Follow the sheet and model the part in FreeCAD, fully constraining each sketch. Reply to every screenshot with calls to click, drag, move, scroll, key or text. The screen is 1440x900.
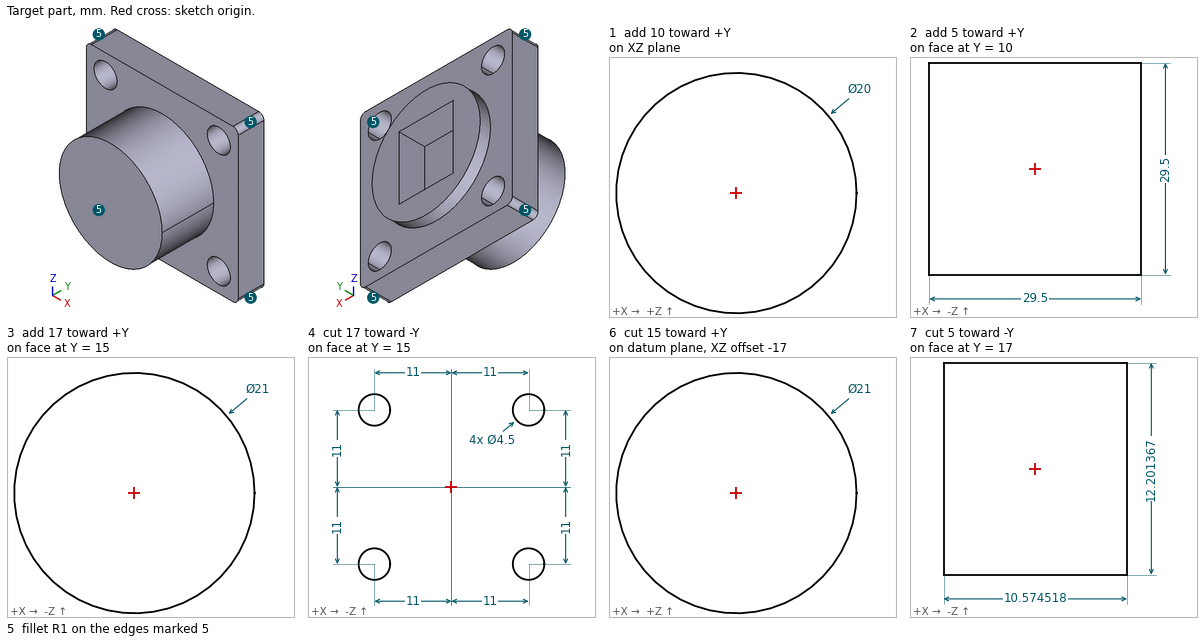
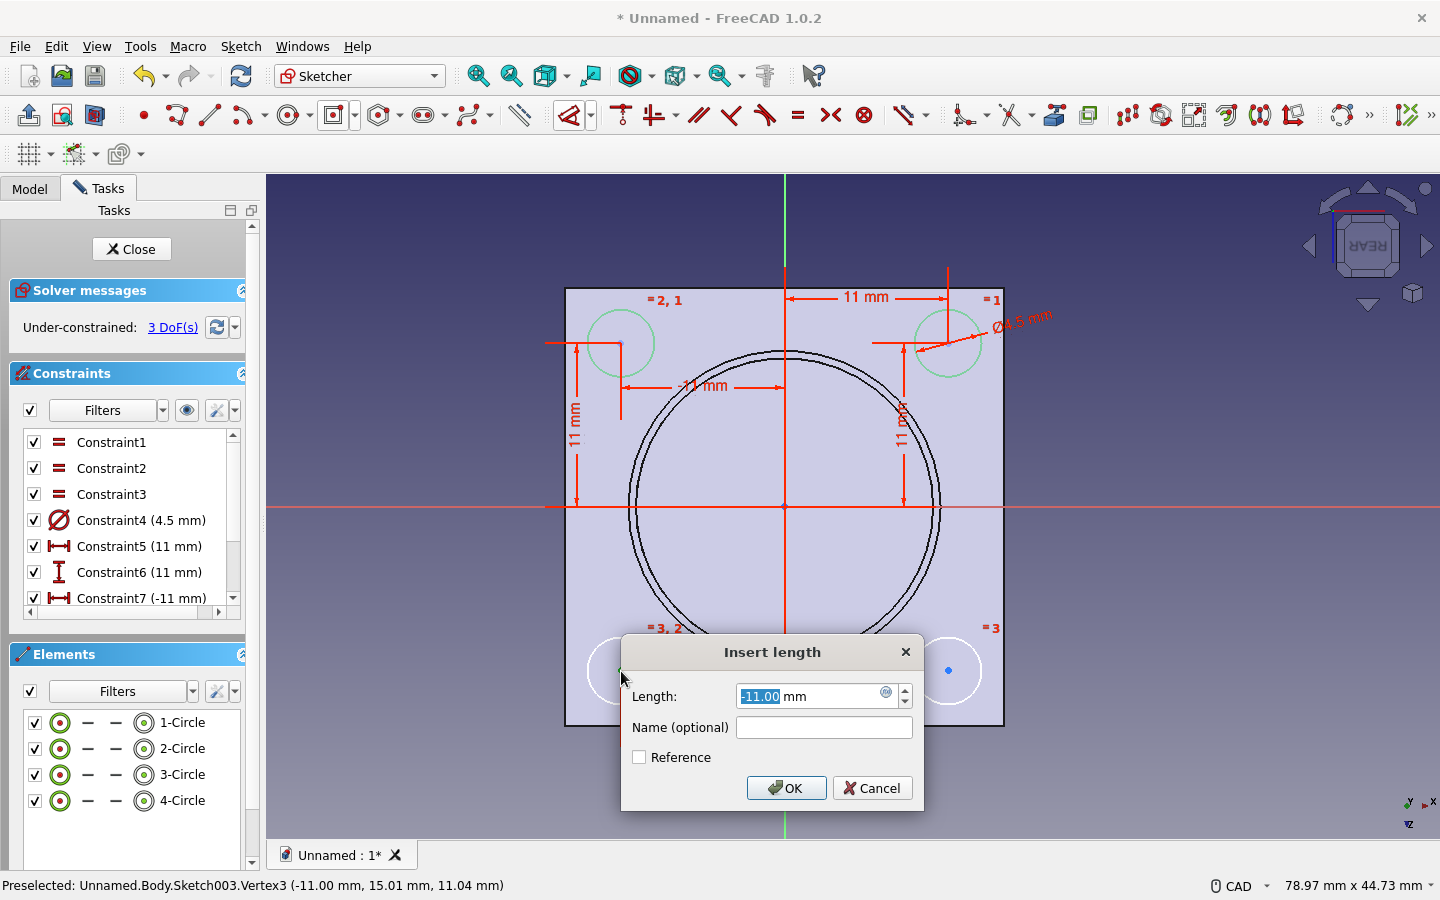
text(-11)
key(Return)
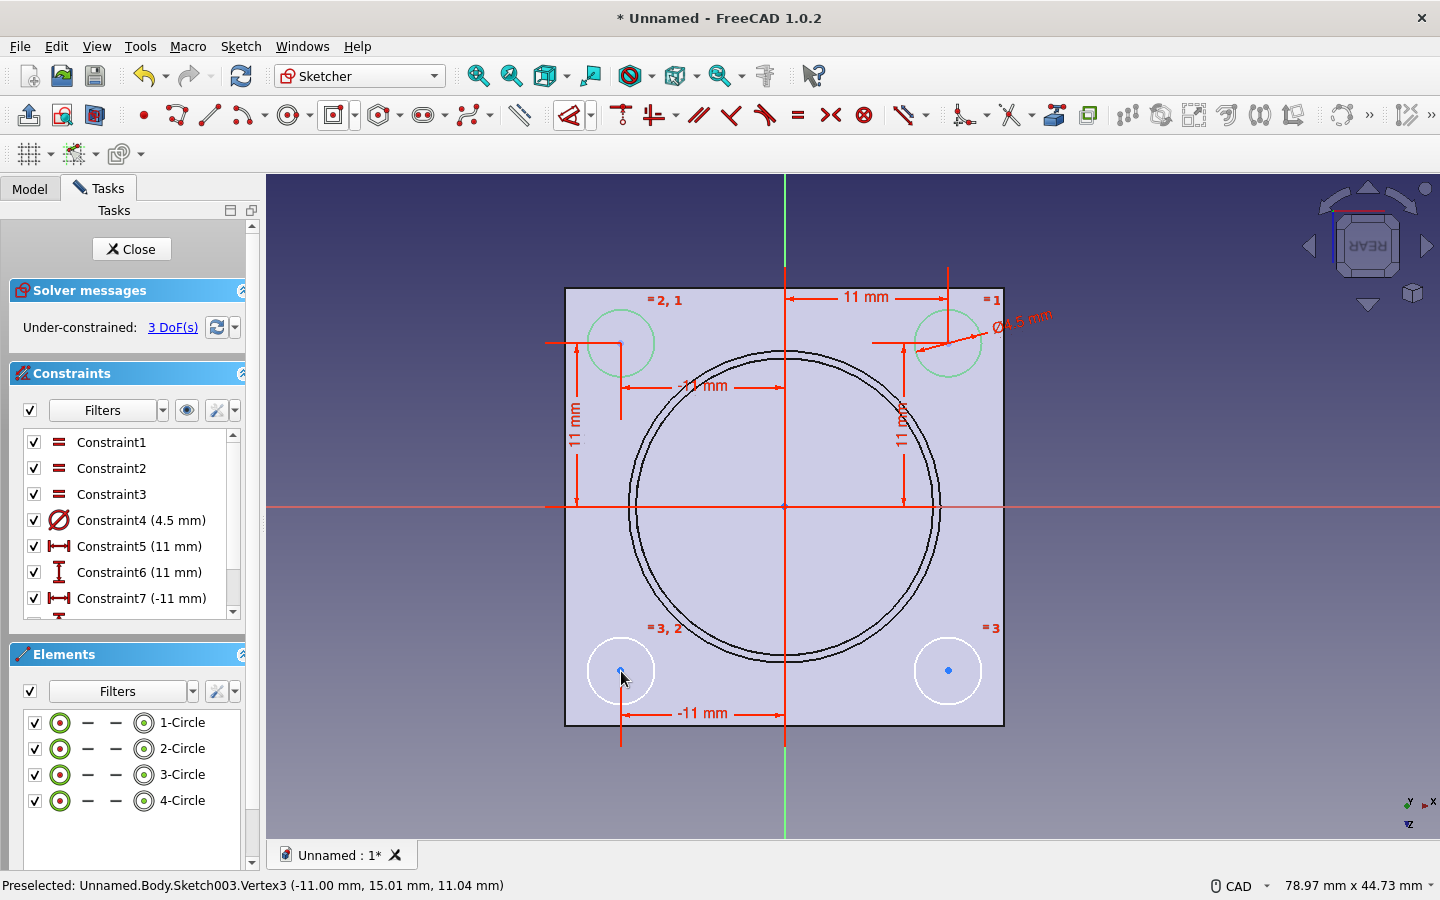
click(621, 671)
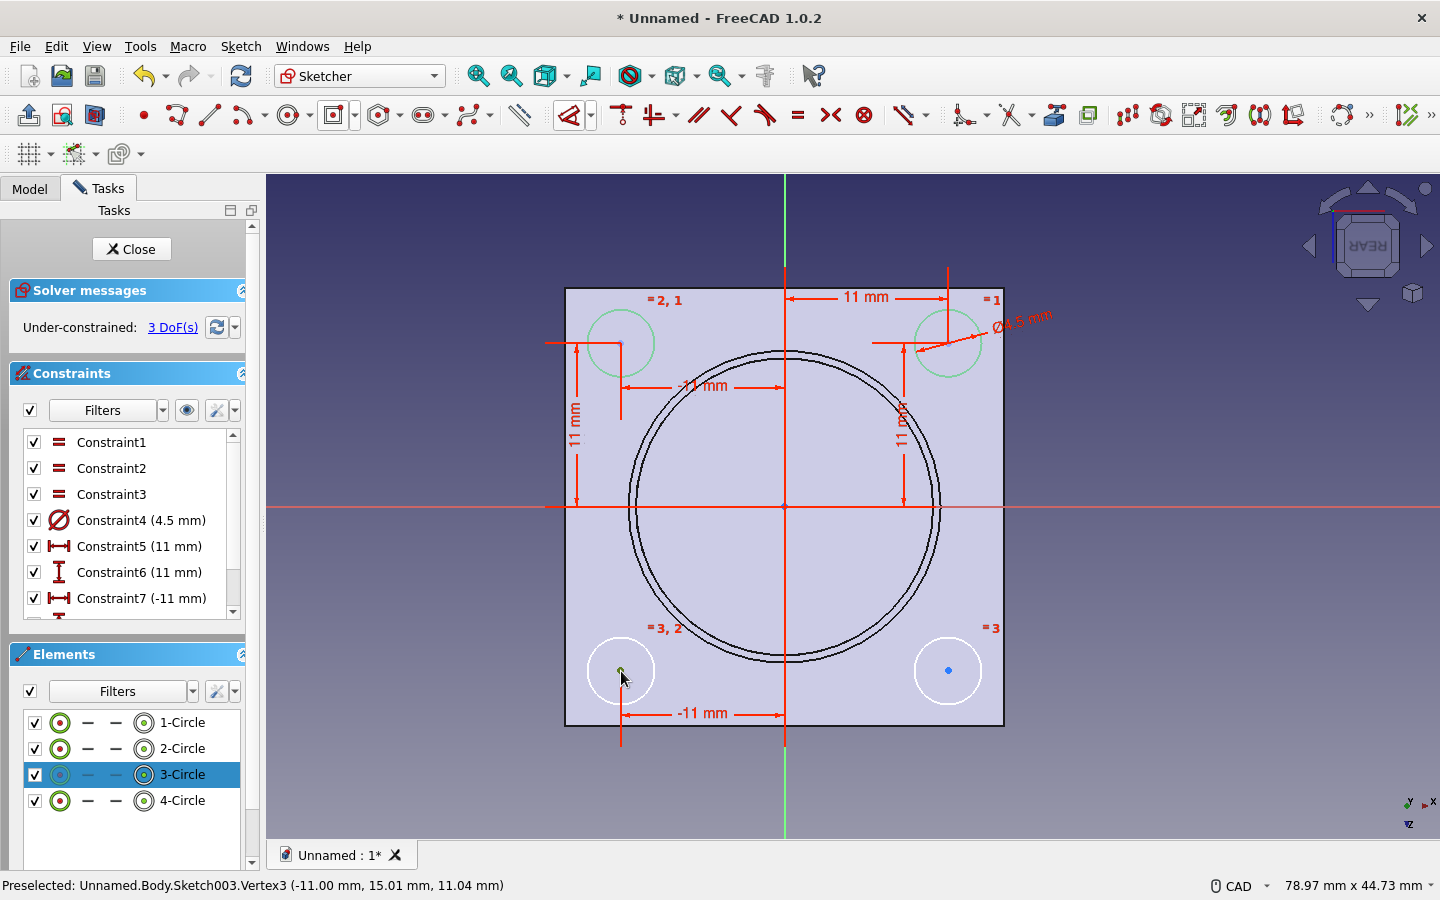
click(590, 116)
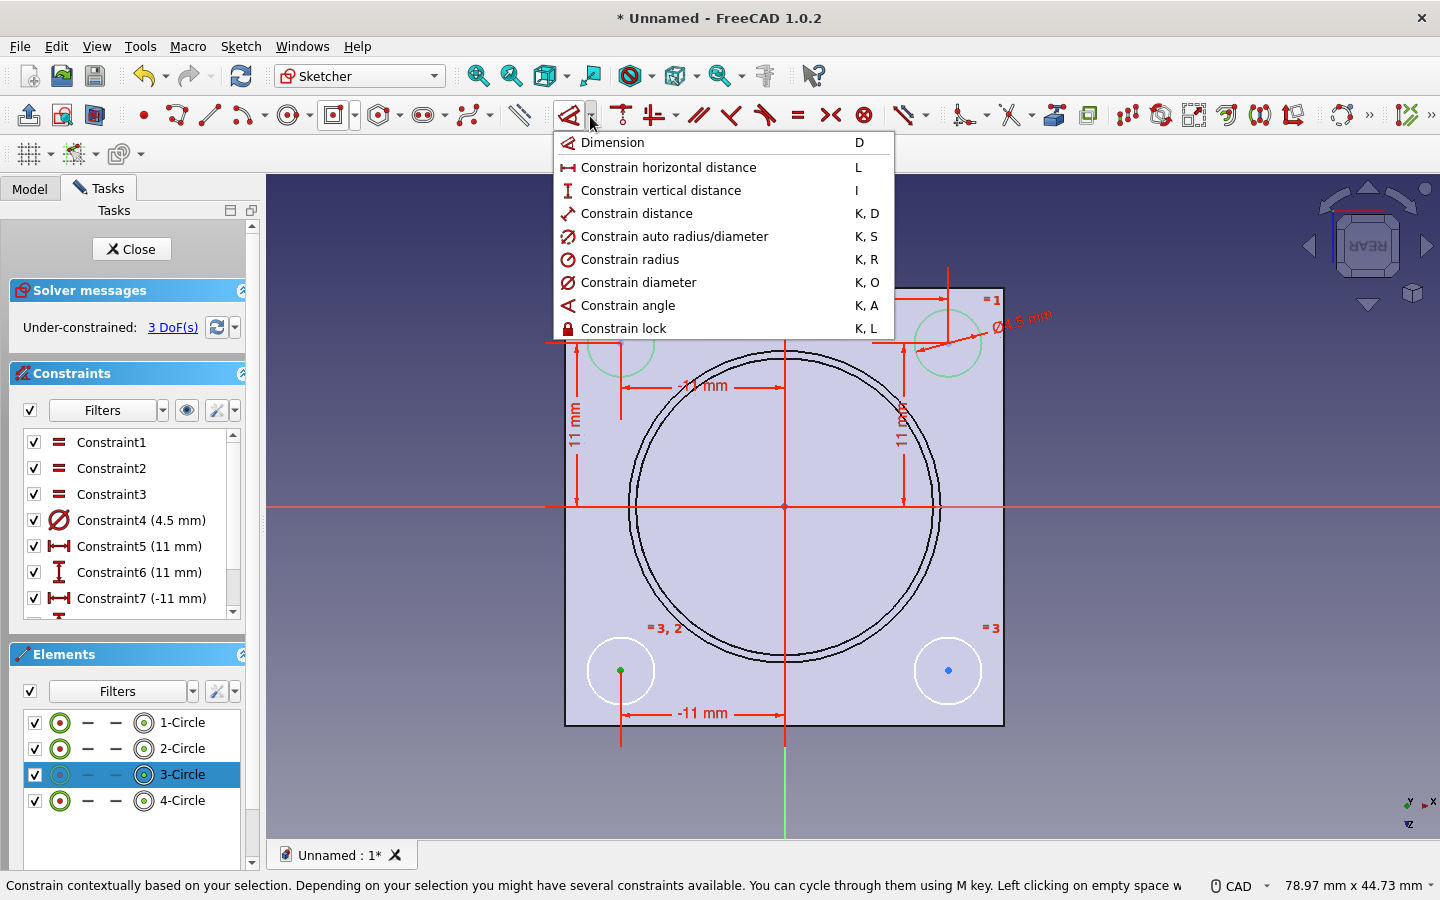
click(724, 190)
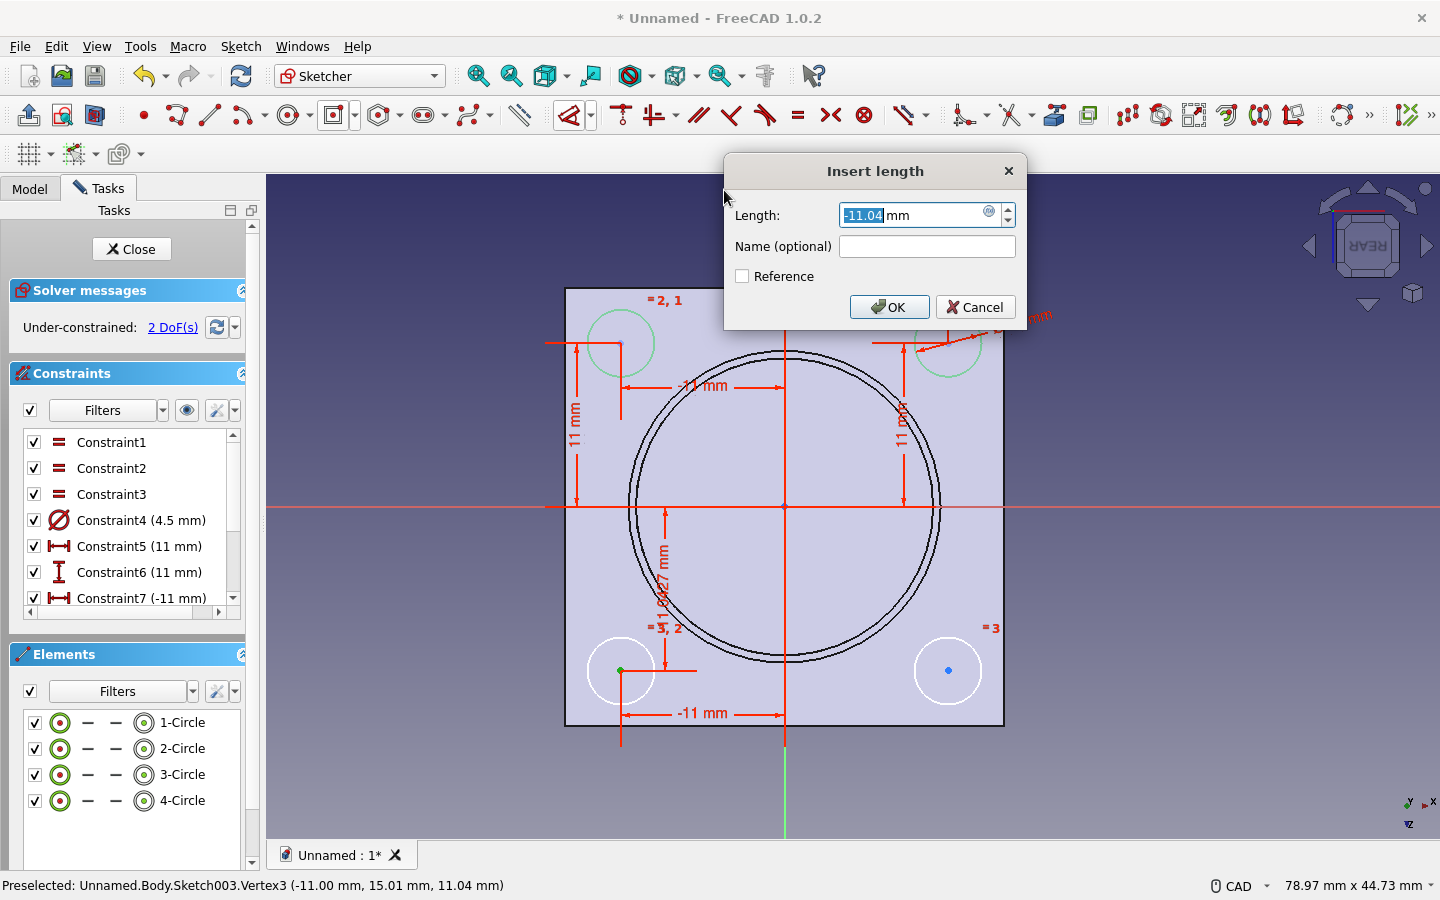
text(-11)
key(Return)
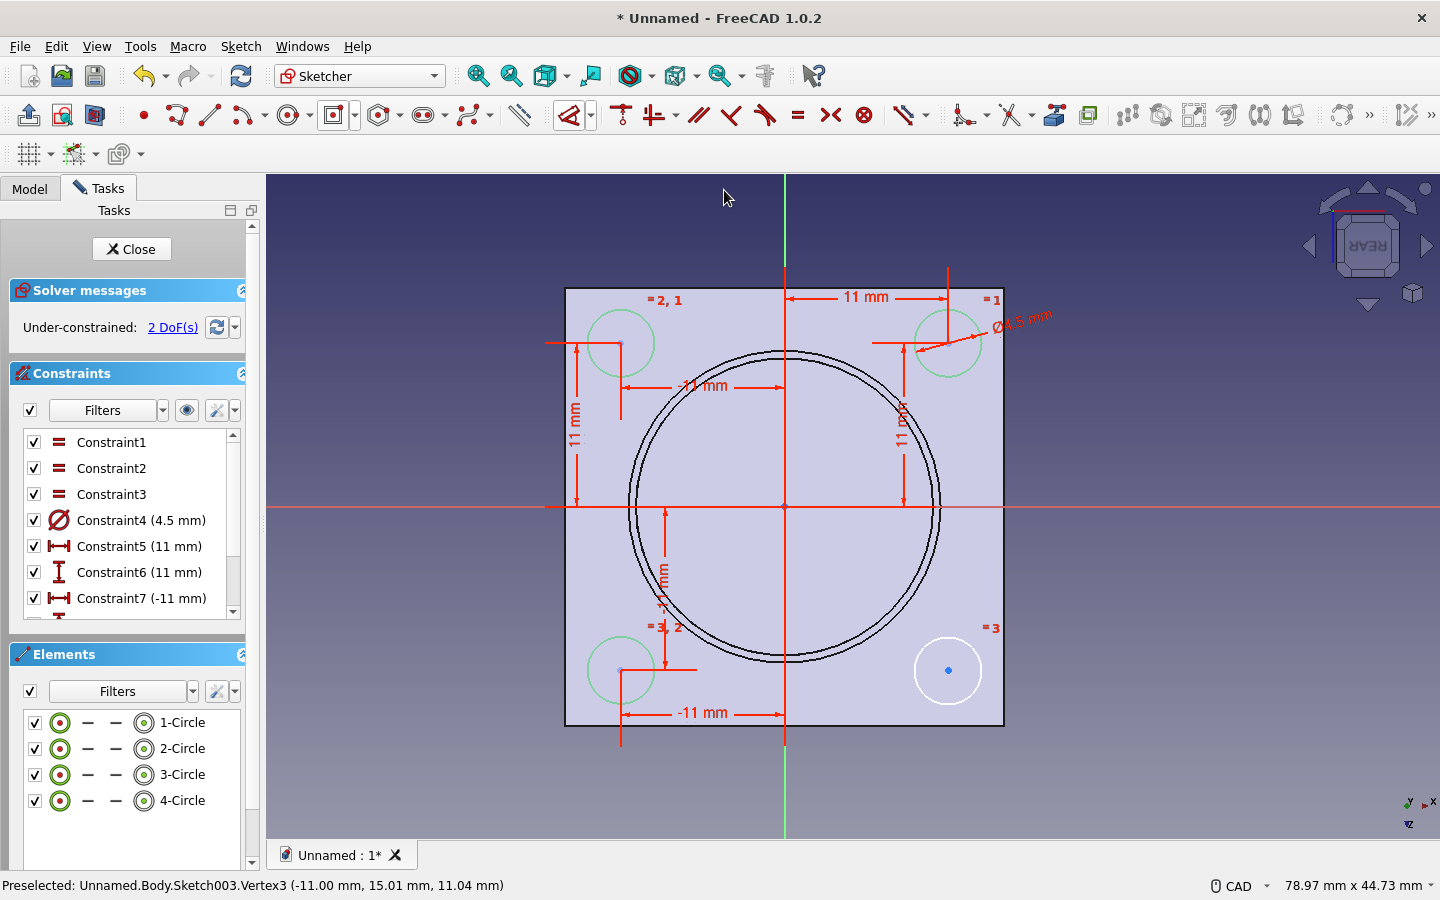
click(948, 671)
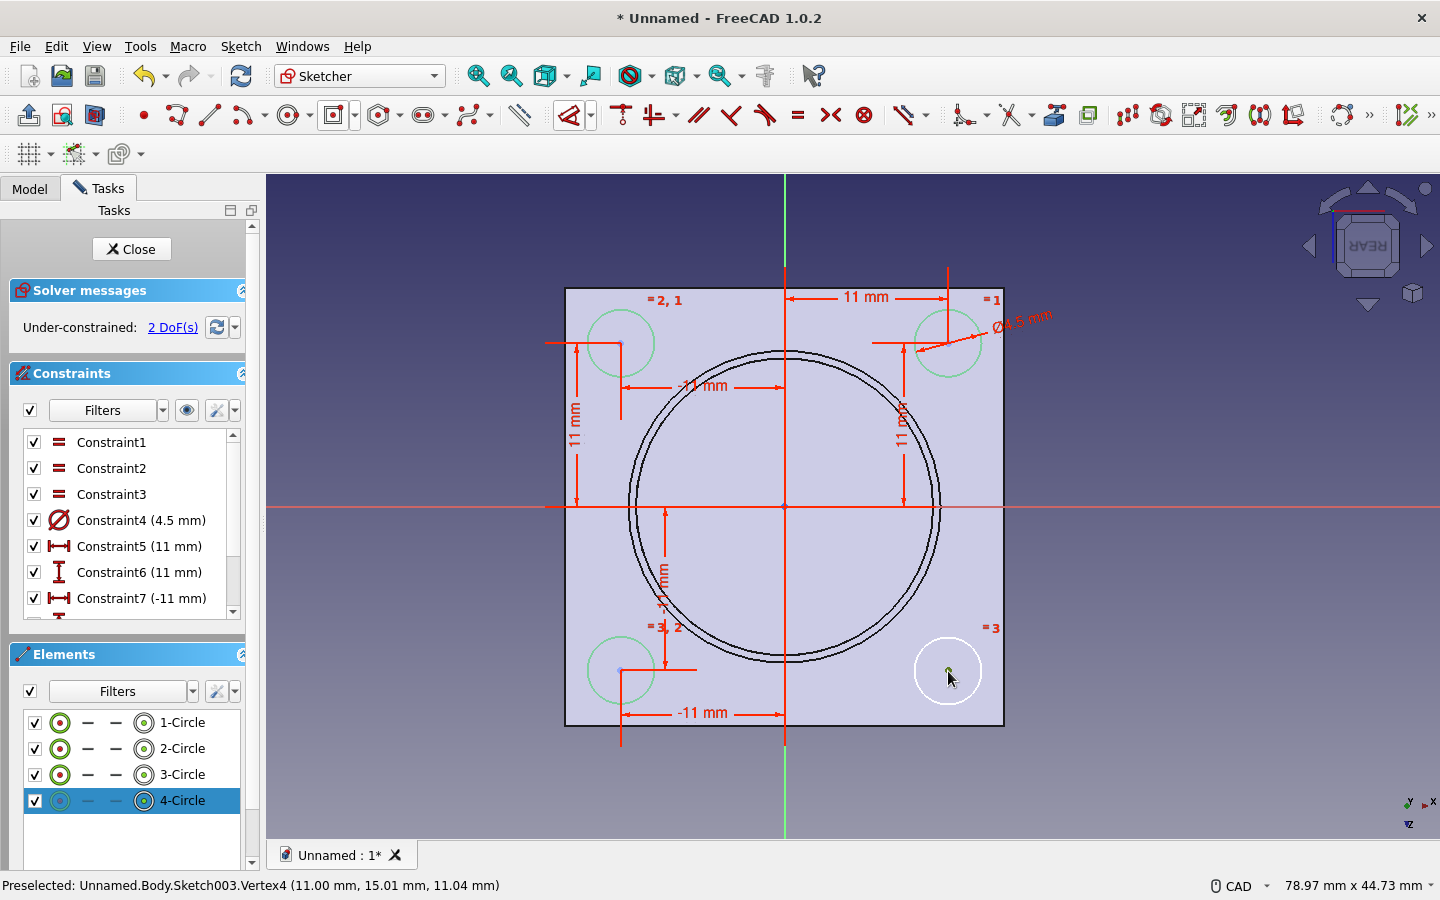
key(l)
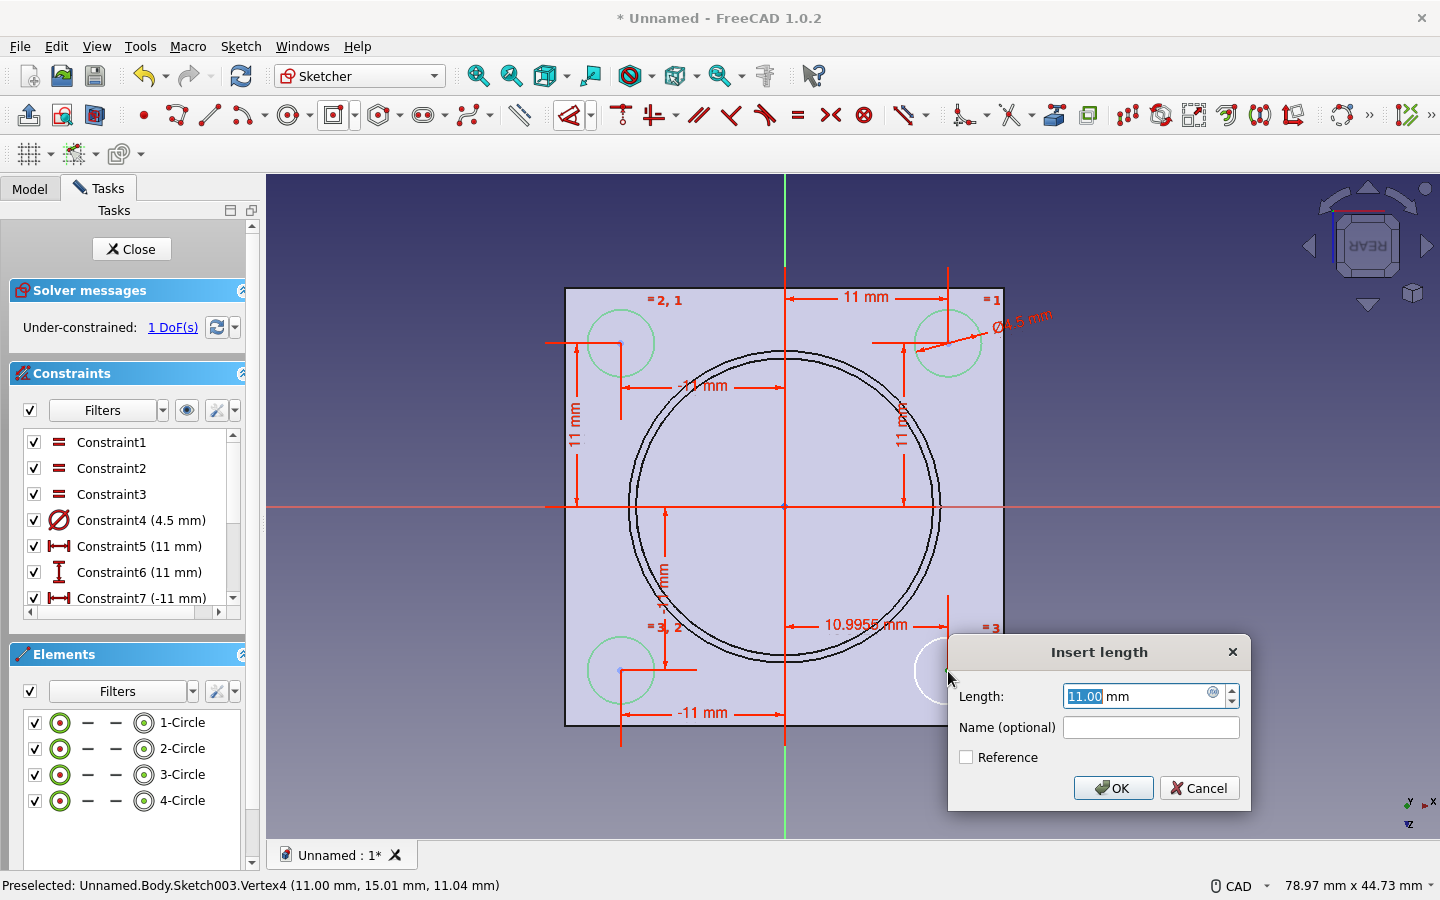
text(11)
key(Return)